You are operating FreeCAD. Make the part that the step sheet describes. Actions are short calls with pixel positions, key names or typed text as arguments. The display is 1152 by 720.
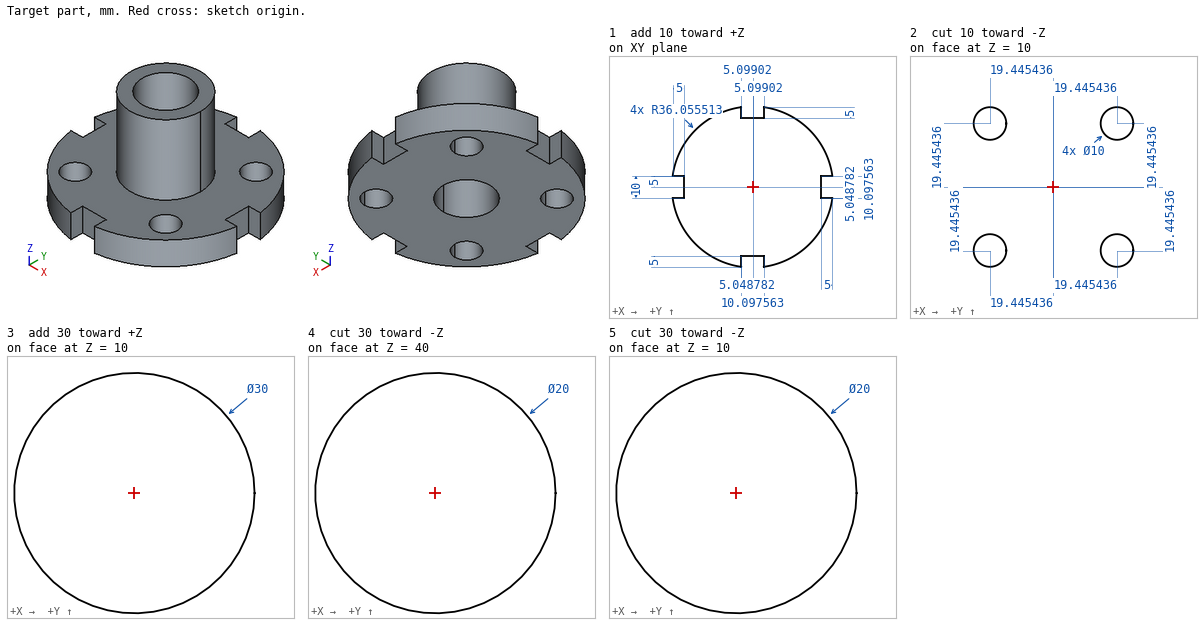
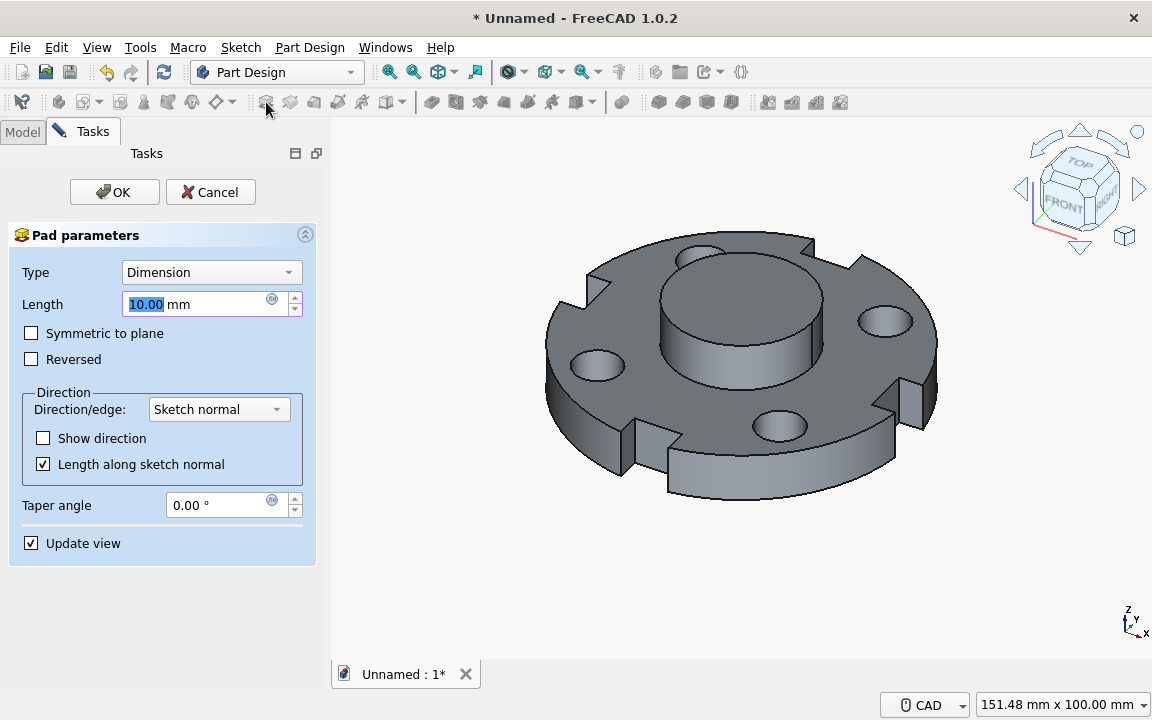
text(30)
key(Tab)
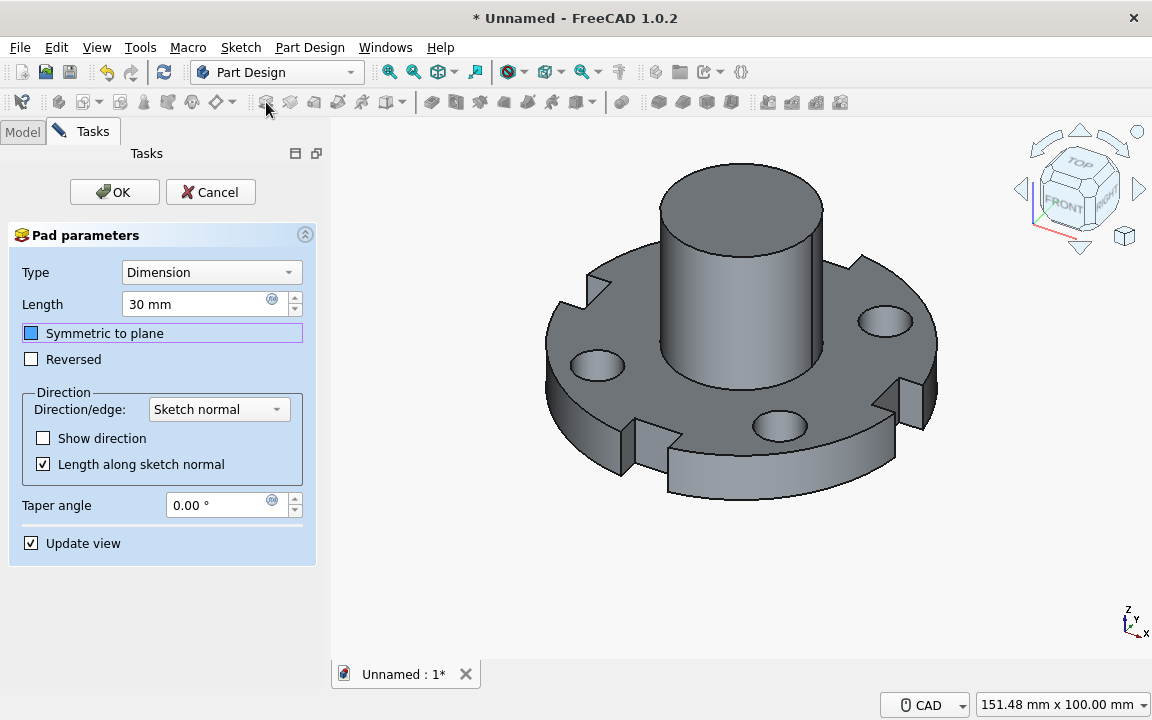
click(115, 192)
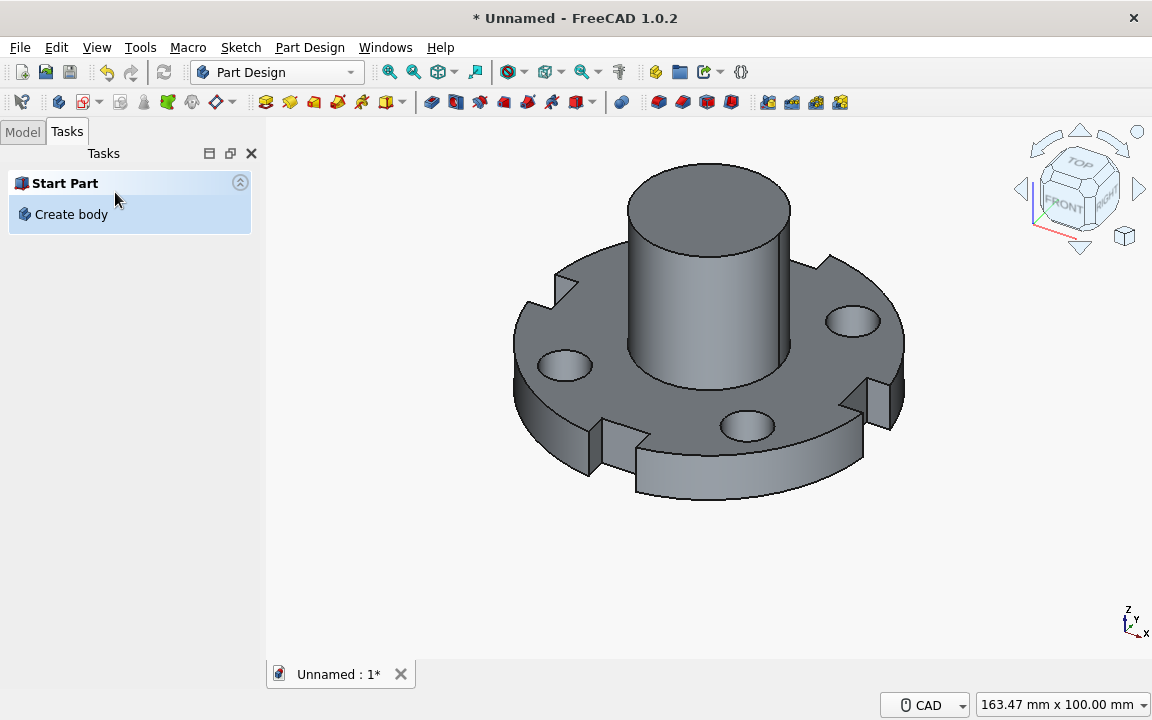
click(390, 72)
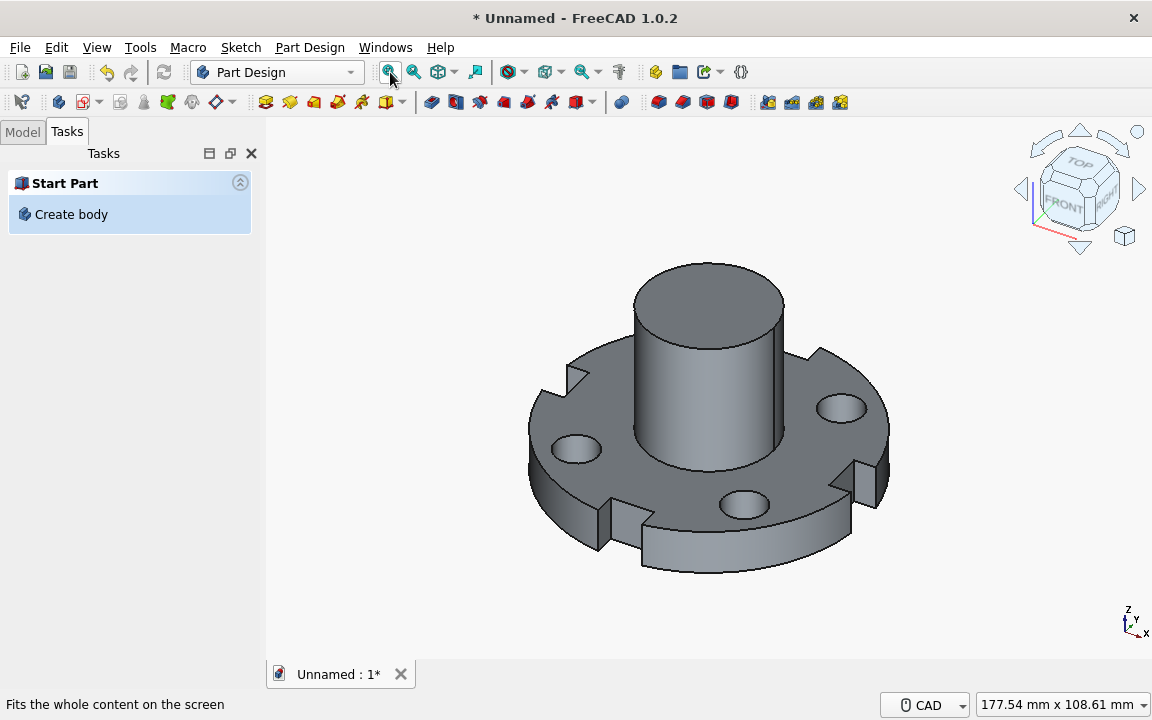
click(709, 305)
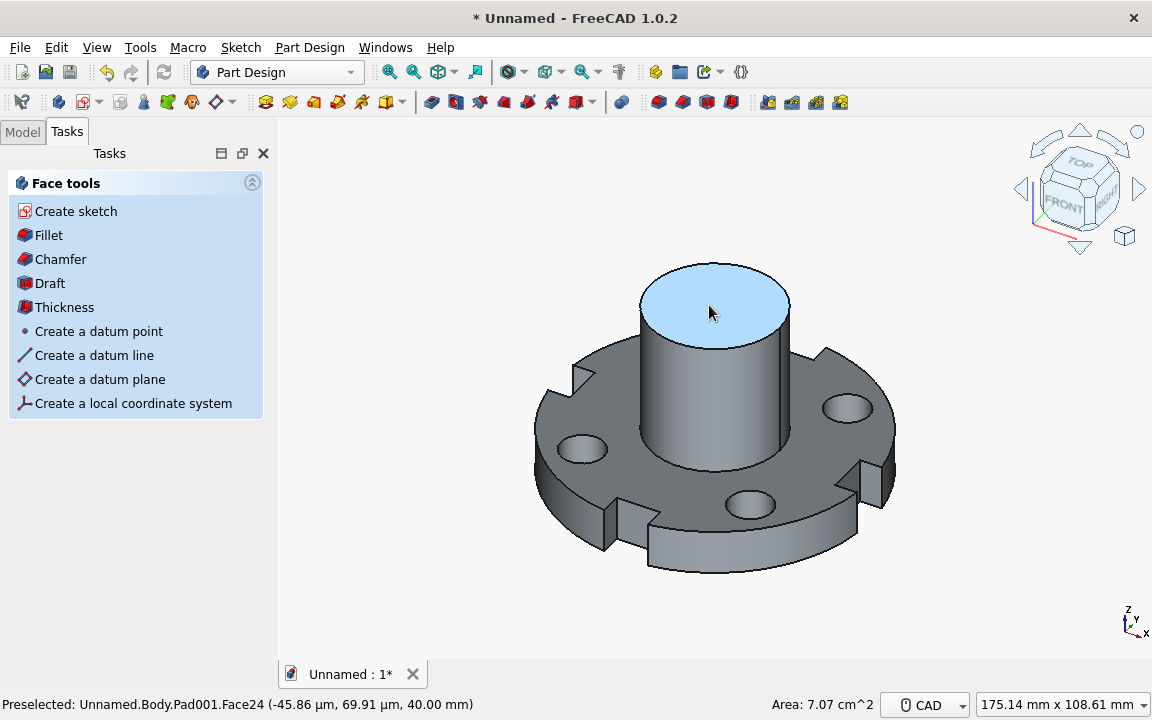
click(84, 102)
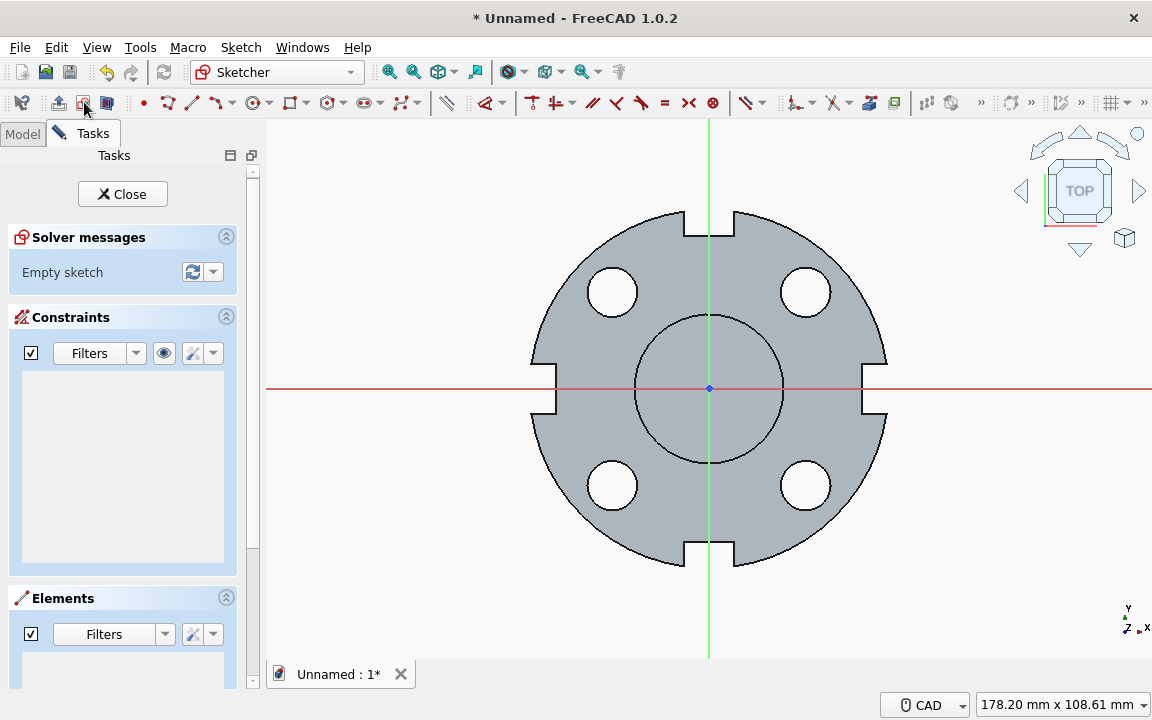
scroll(739, 389, up, 6)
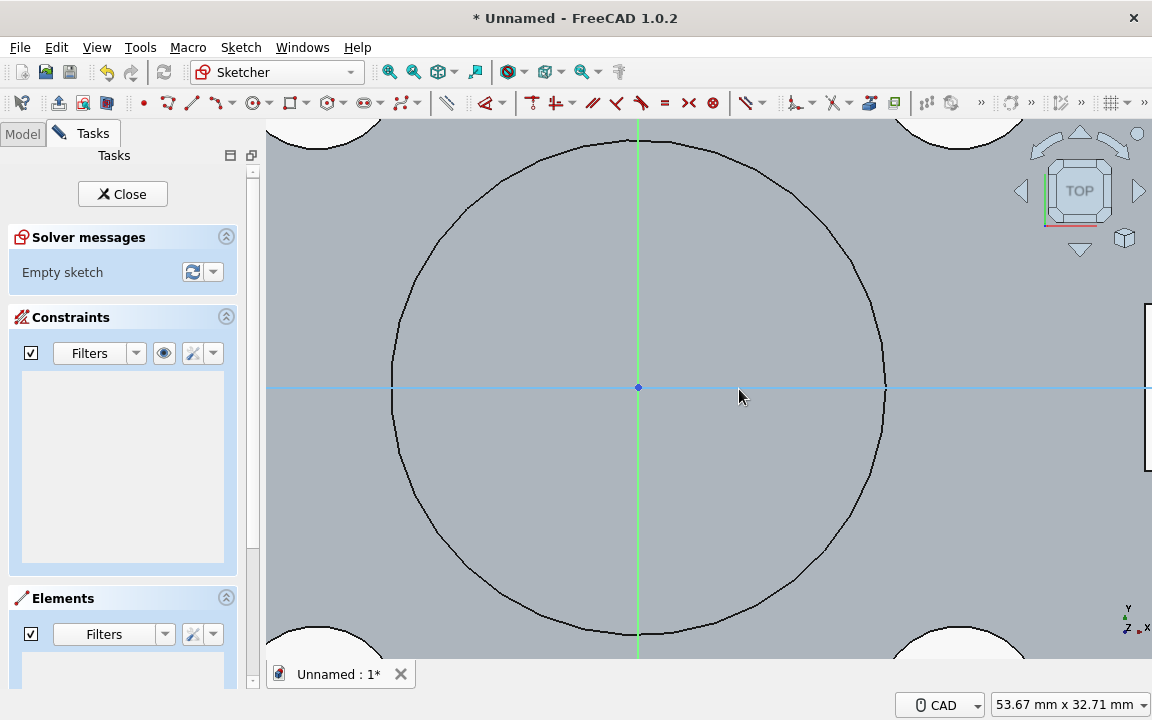
click(254, 104)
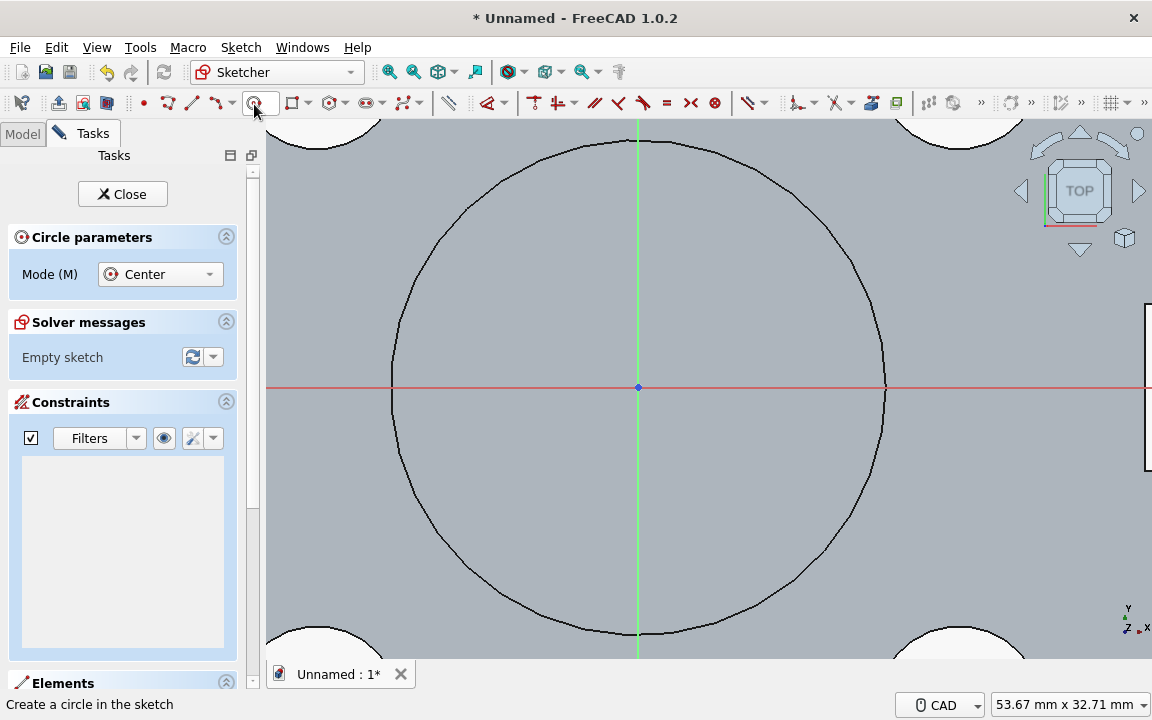
click(638, 388)
move(755, 271)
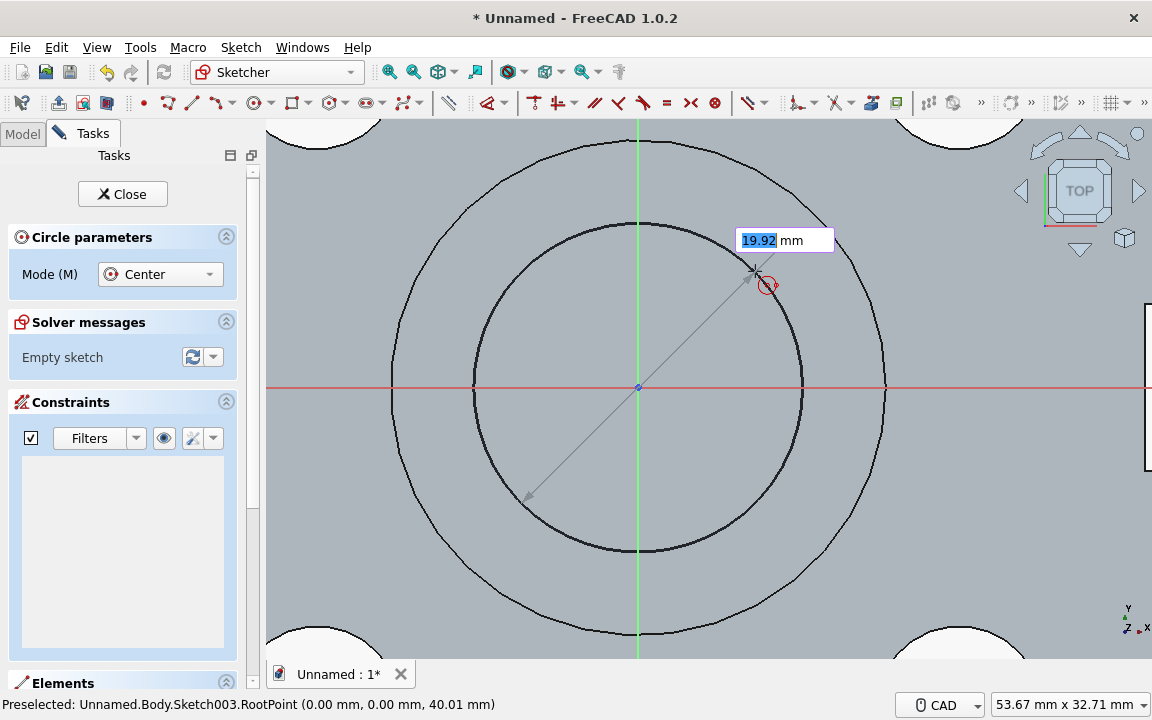
text(20)
key(Return)
key(Escape)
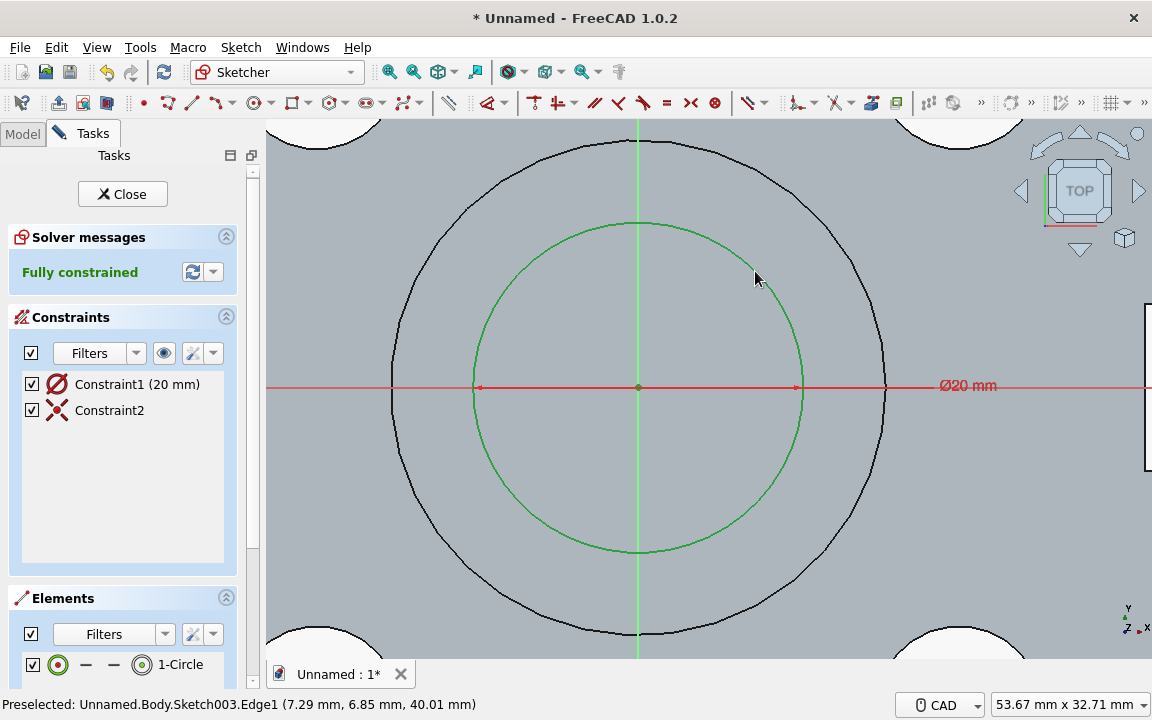
click(123, 194)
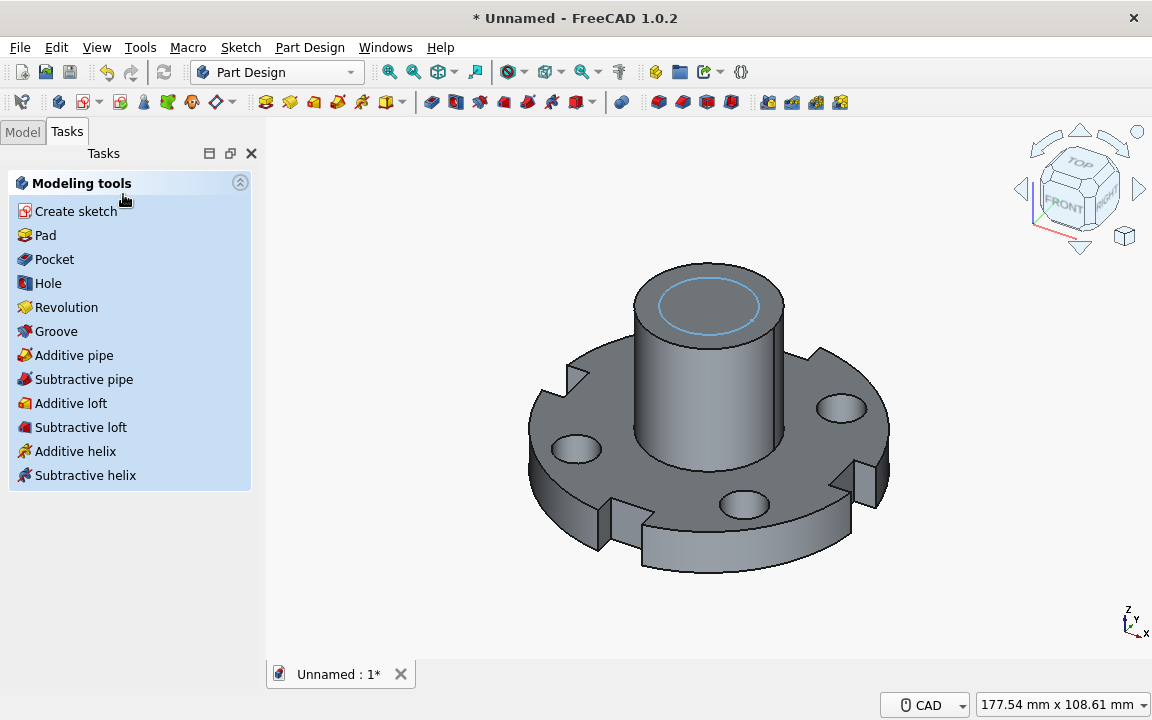
click(432, 102)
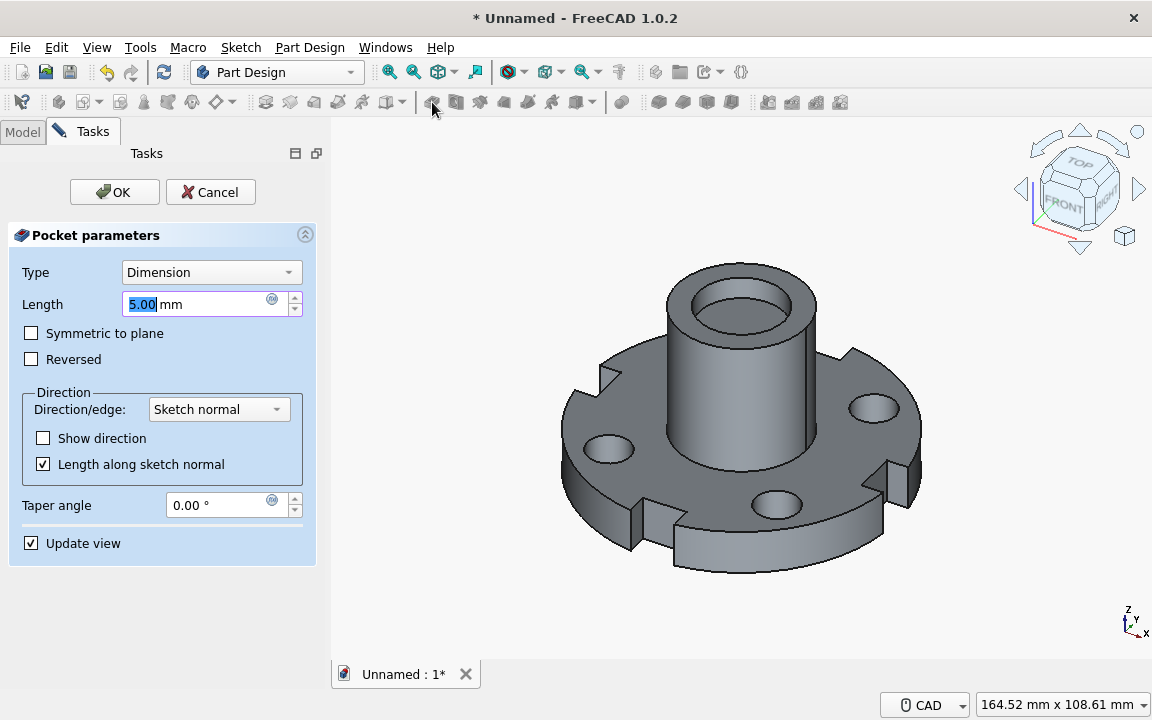
text(30)
key(Tab)